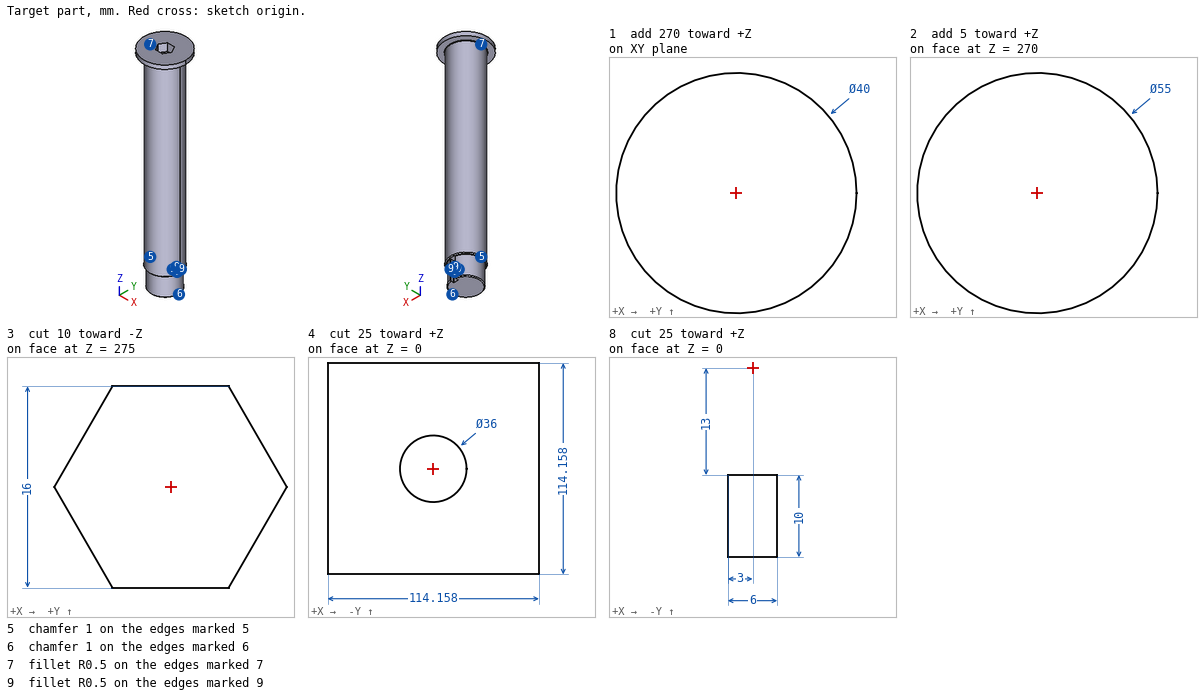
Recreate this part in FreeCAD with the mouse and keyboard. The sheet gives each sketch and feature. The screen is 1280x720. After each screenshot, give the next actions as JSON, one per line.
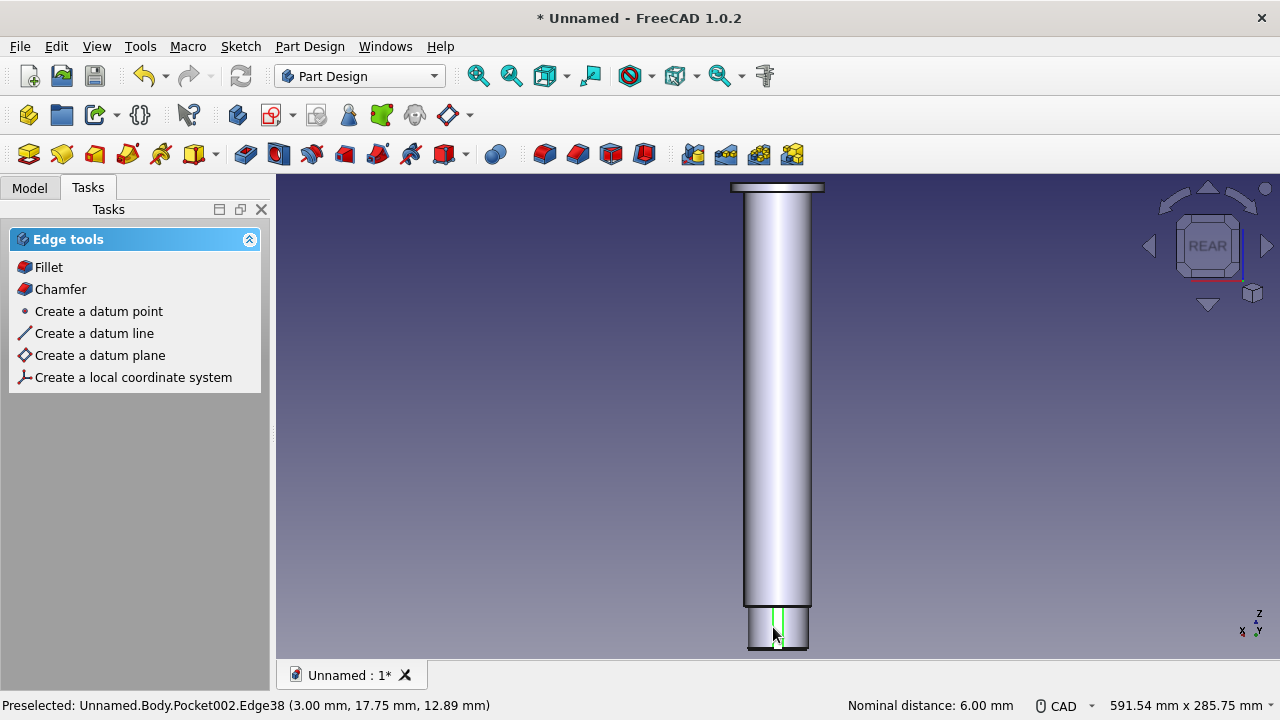
{"action": "key", "text": "6"}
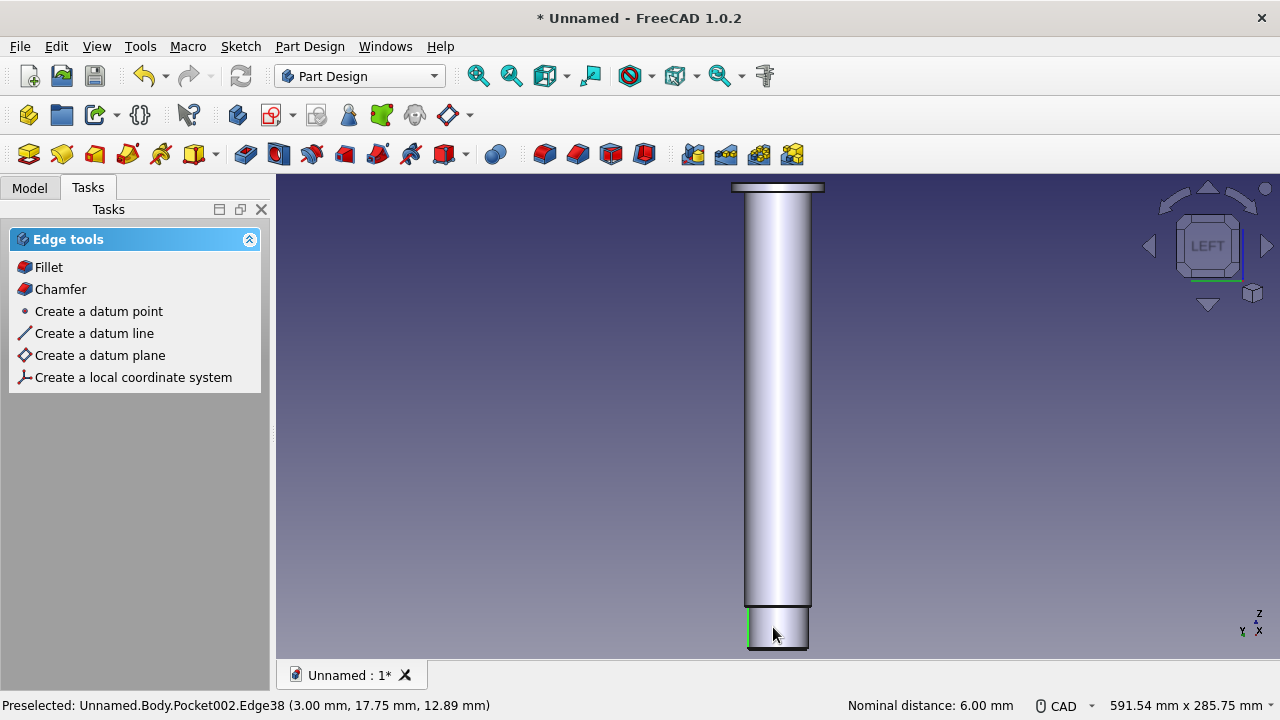
{"action": "key", "text": "v 3"}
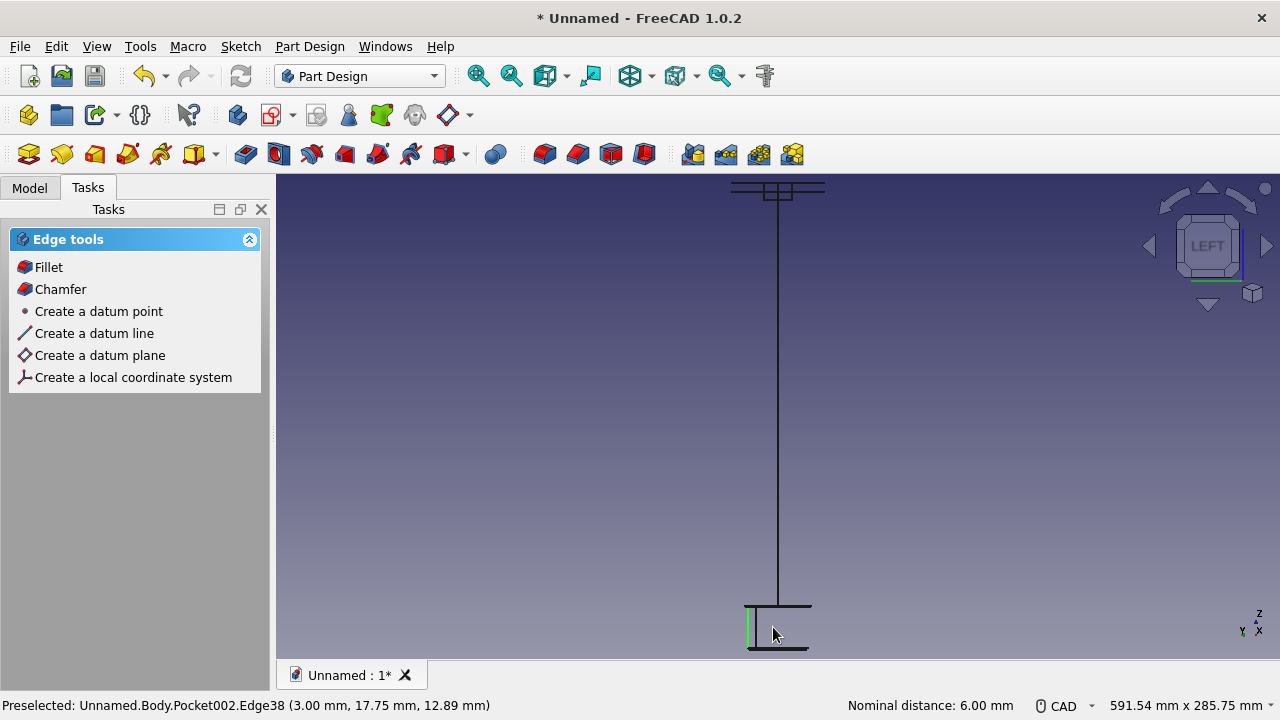
{"action": "key", "text": "0"}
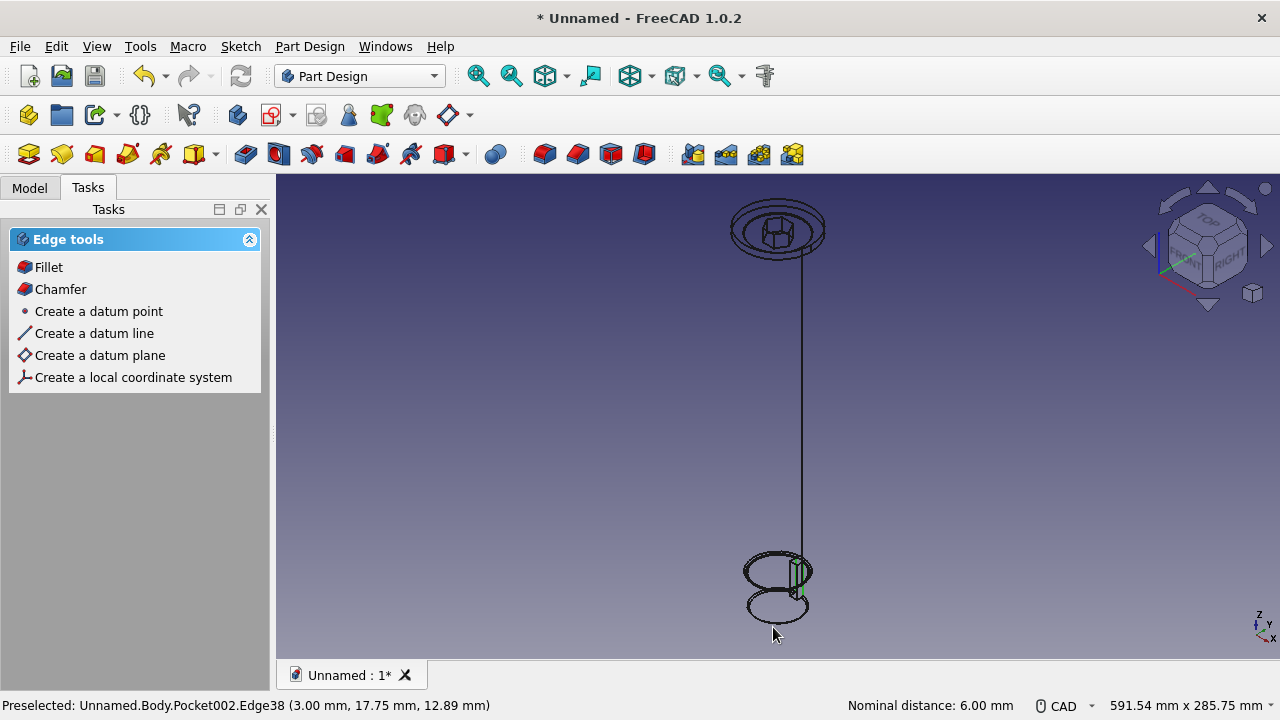
{"action": "left_click", "coordinate": [797, 595], "text": "ctrl"}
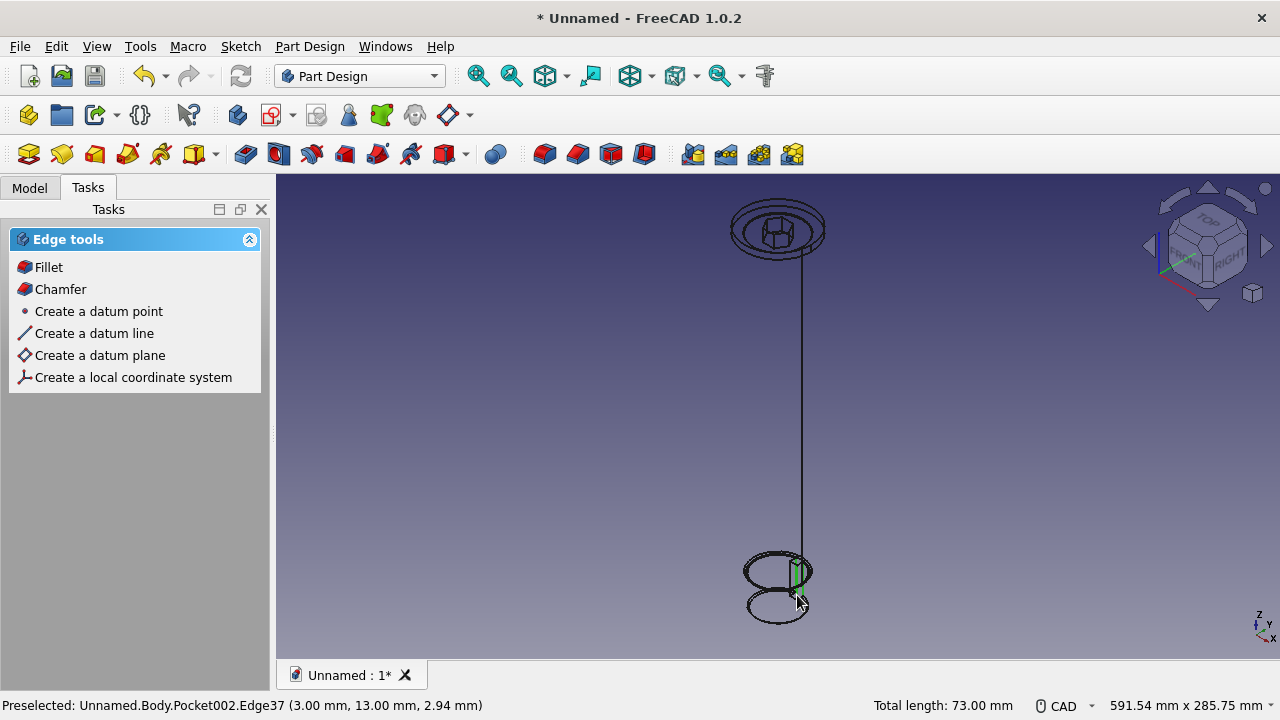
{"action": "left_click", "coordinate": [790, 578], "text": "ctrl"}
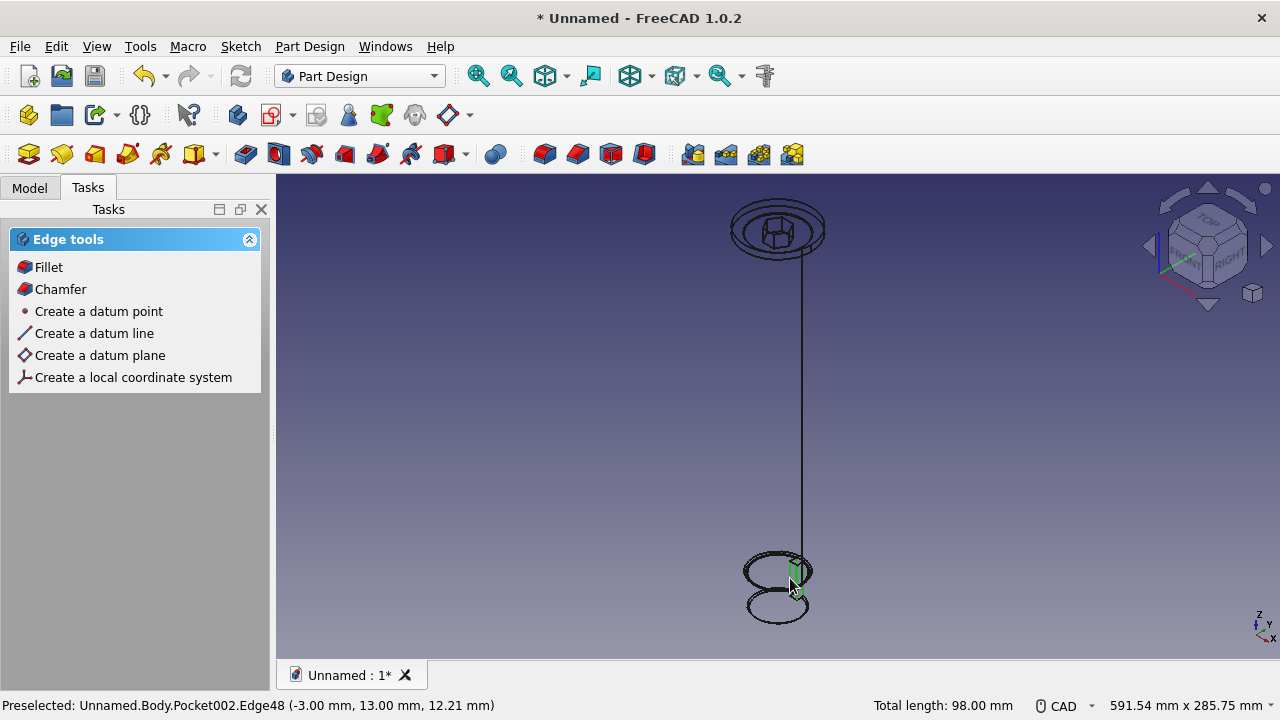
{"action": "key", "text": "v 1"}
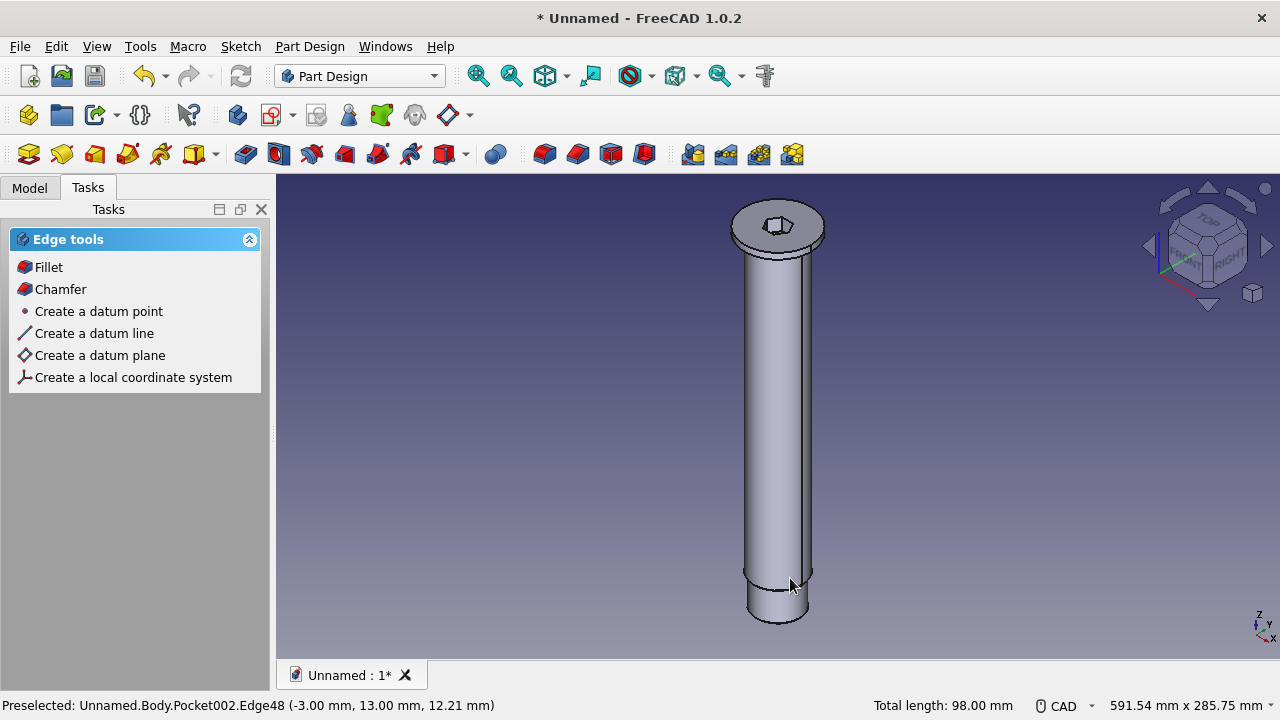
{"action": "left_click", "coordinate": [545, 154]}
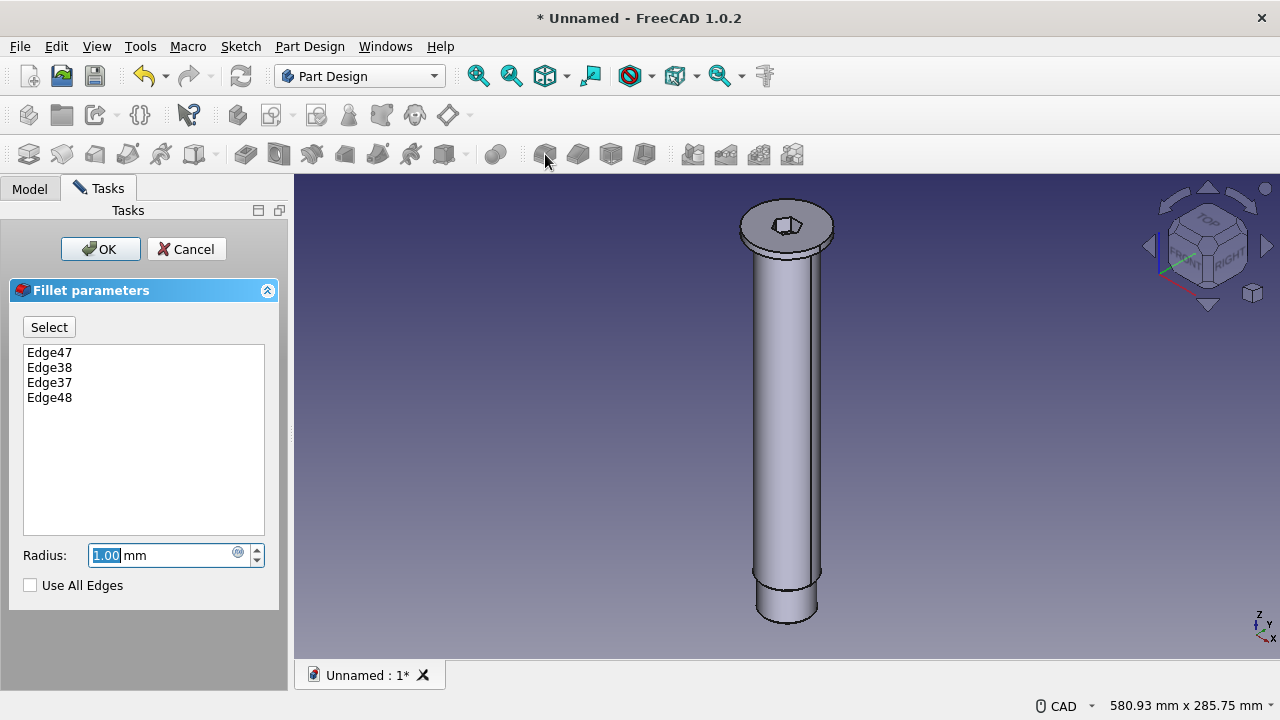
{"action": "type", "text": "0.5"}
{"action": "key", "text": "Tab"}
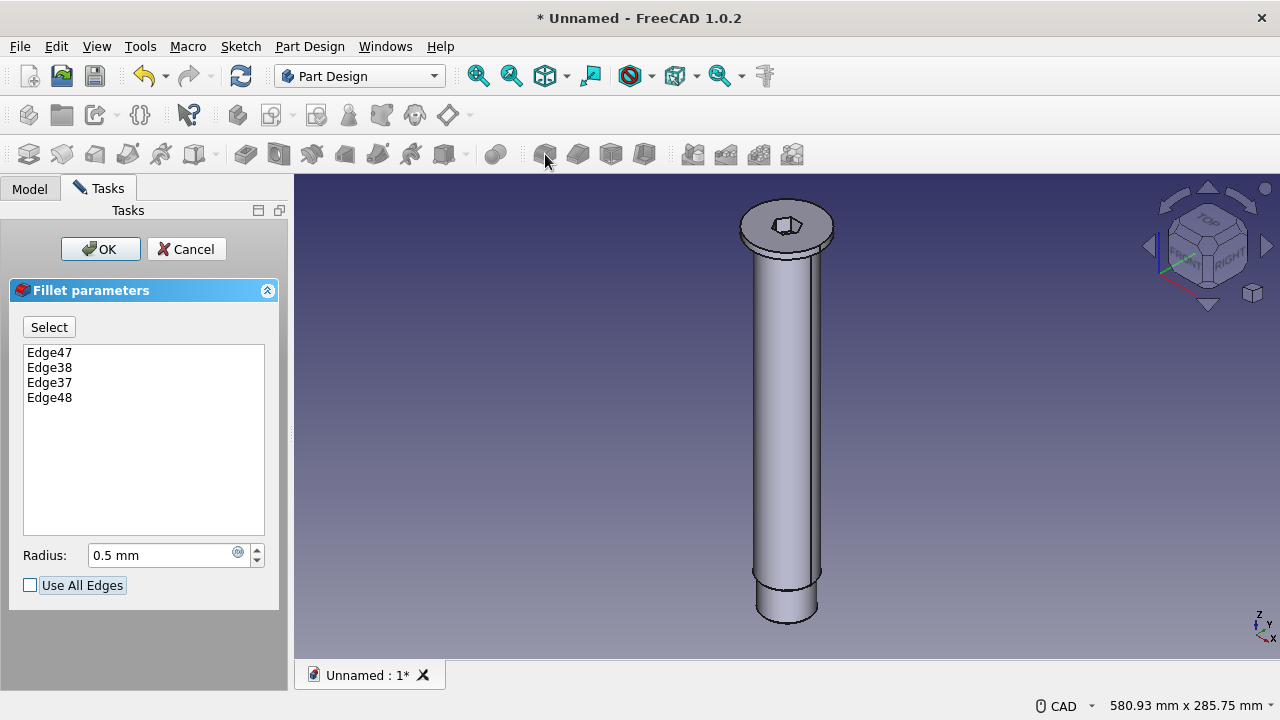
{"action": "left_click", "coordinate": [101, 249]}